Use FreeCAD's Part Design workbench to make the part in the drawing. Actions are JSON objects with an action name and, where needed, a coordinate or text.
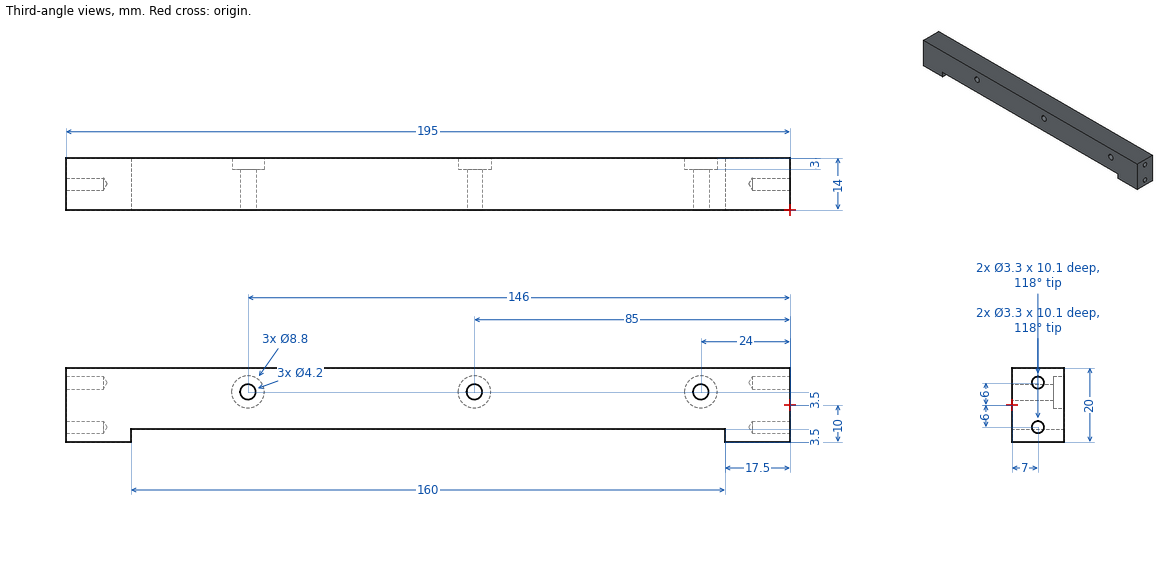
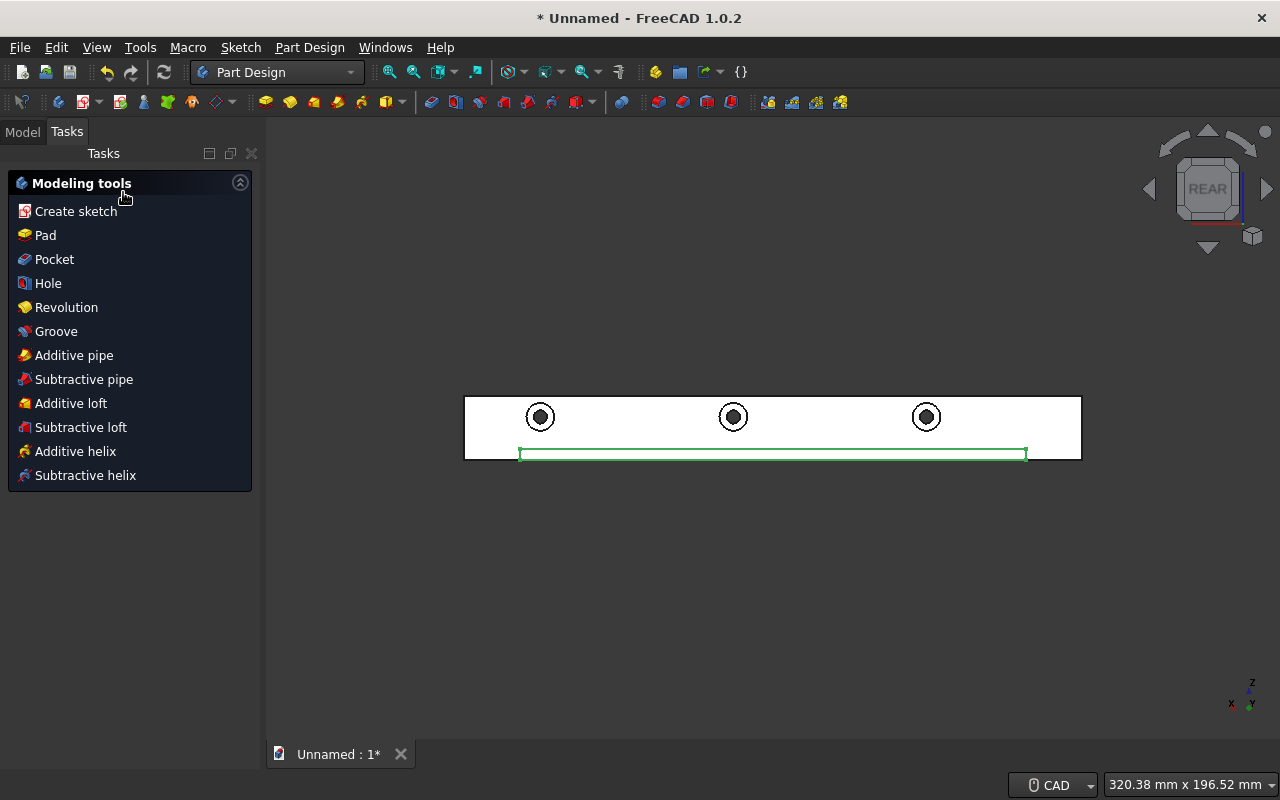
{"action": "left_click", "coordinate": [432, 102]}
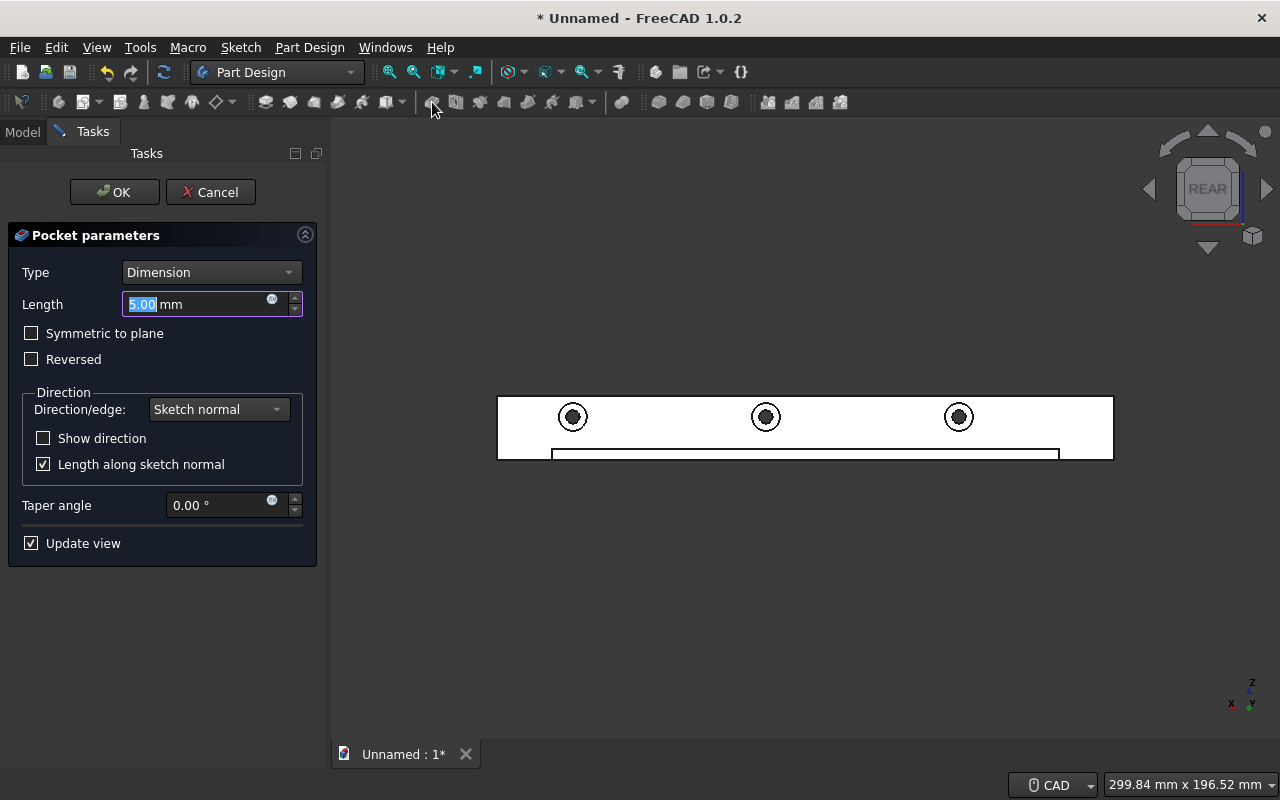
{"action": "left_click", "coordinate": [212, 272]}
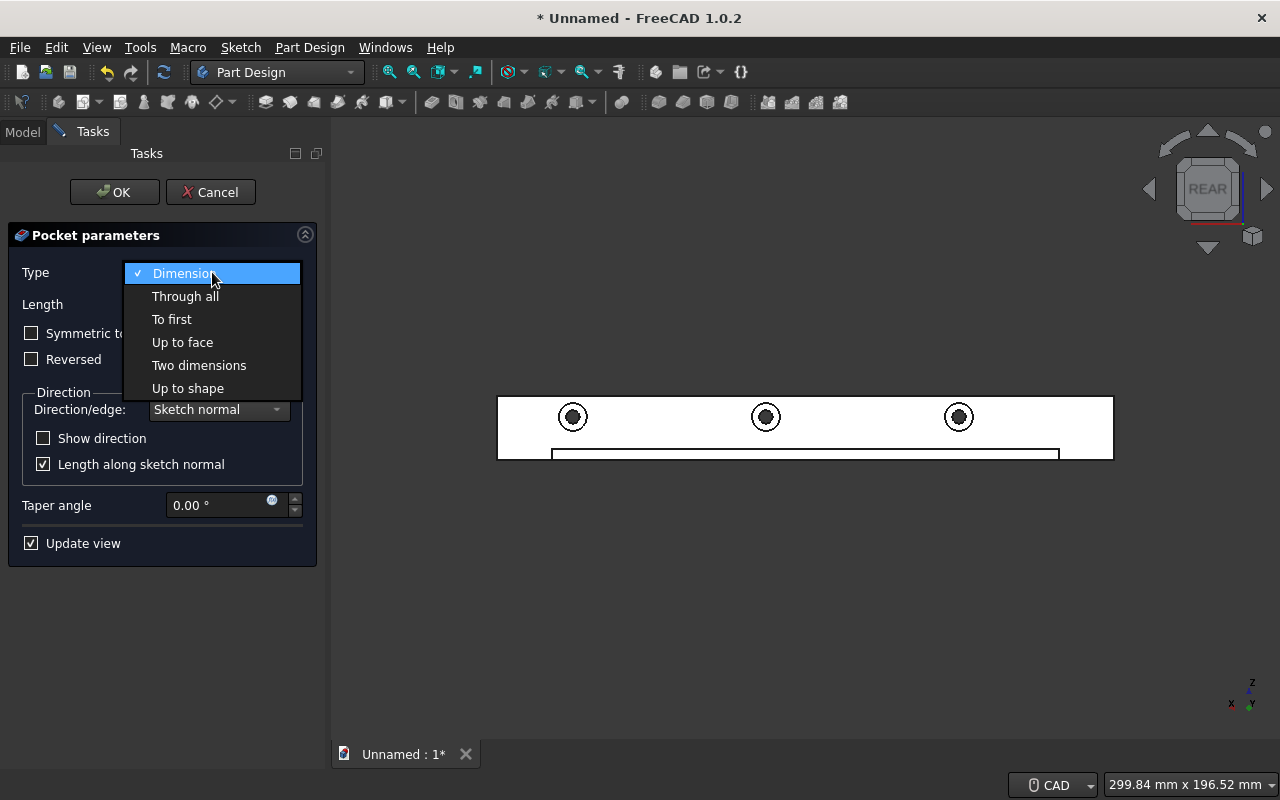
{"action": "left_click", "coordinate": [212, 296]}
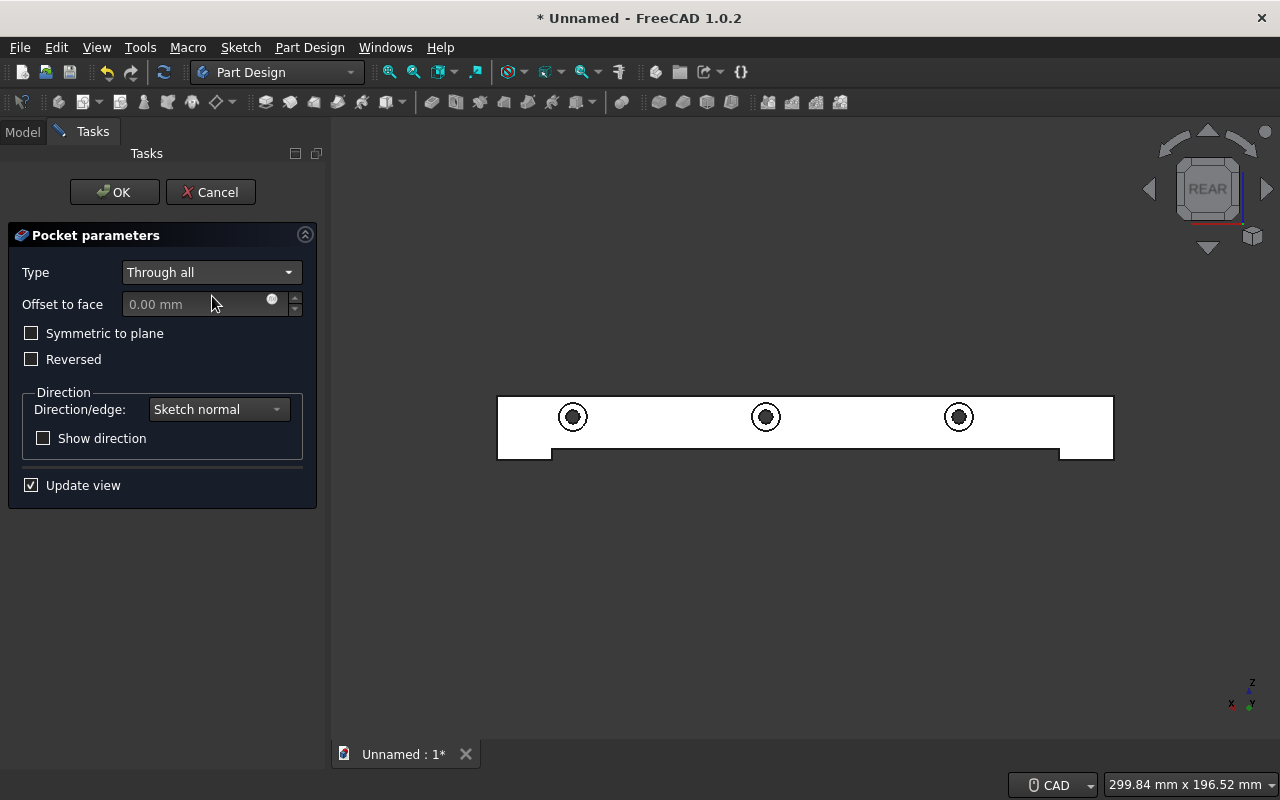
{"action": "left_click", "coordinate": [115, 192]}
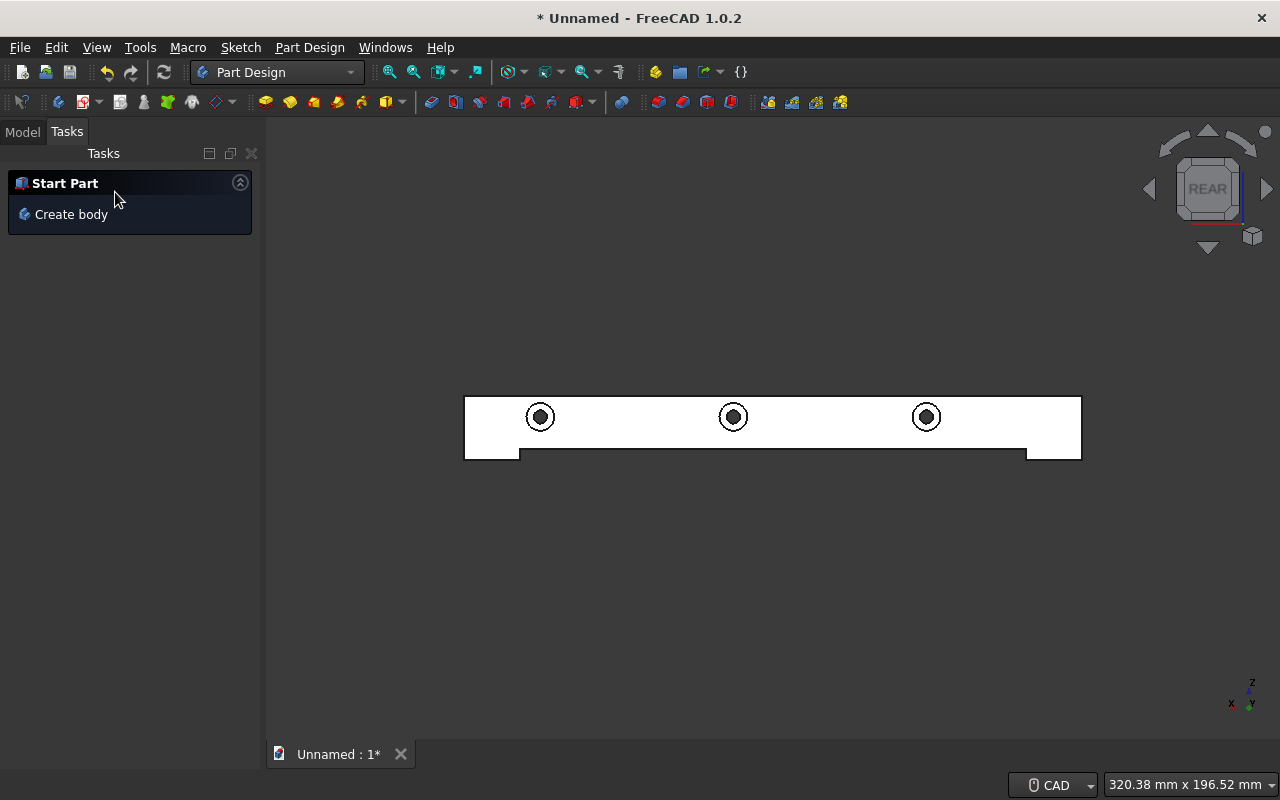
{"action": "key", "text": "0"}